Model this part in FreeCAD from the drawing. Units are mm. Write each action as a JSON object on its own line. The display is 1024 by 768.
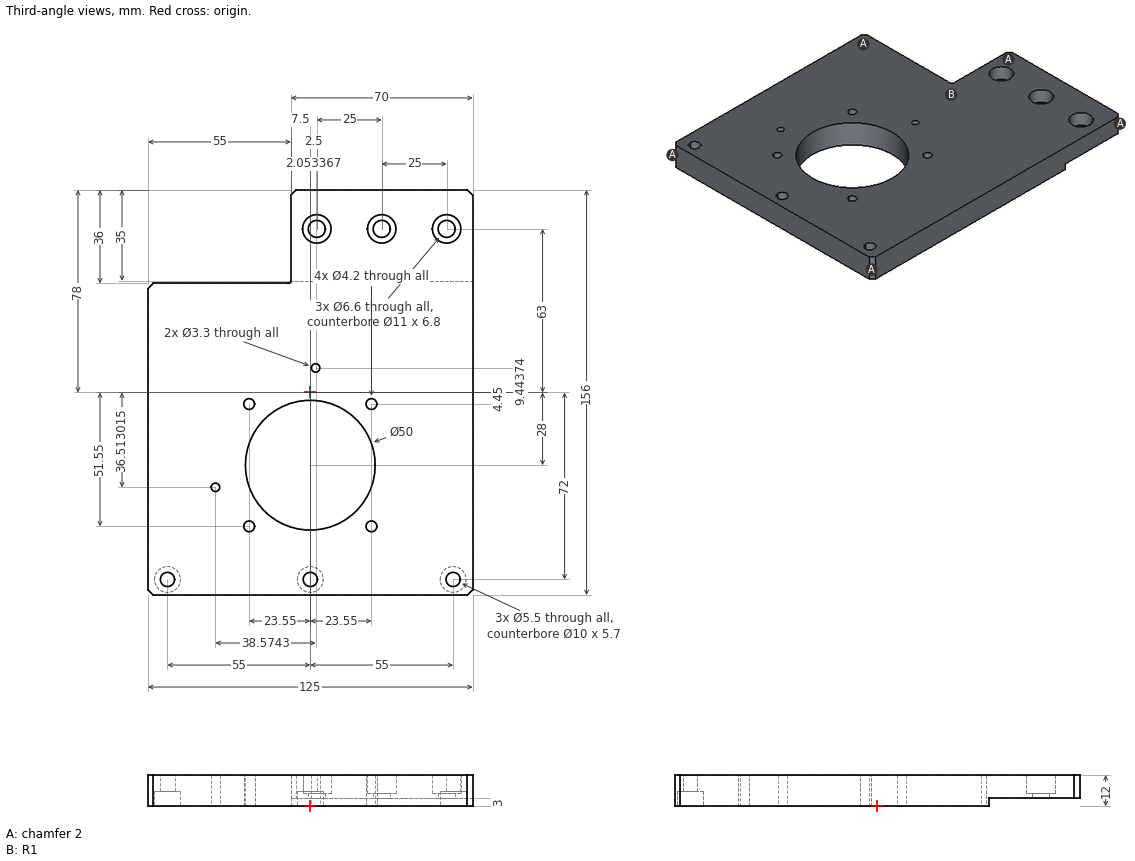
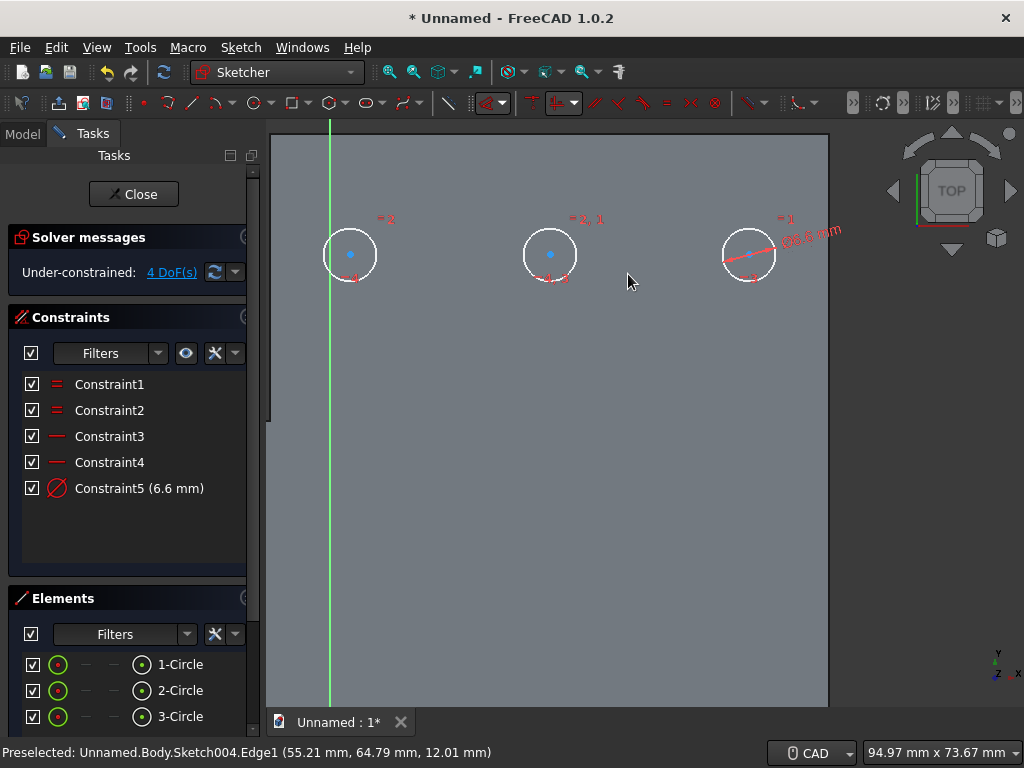
{"action": "left_click", "coordinate": [749, 255]}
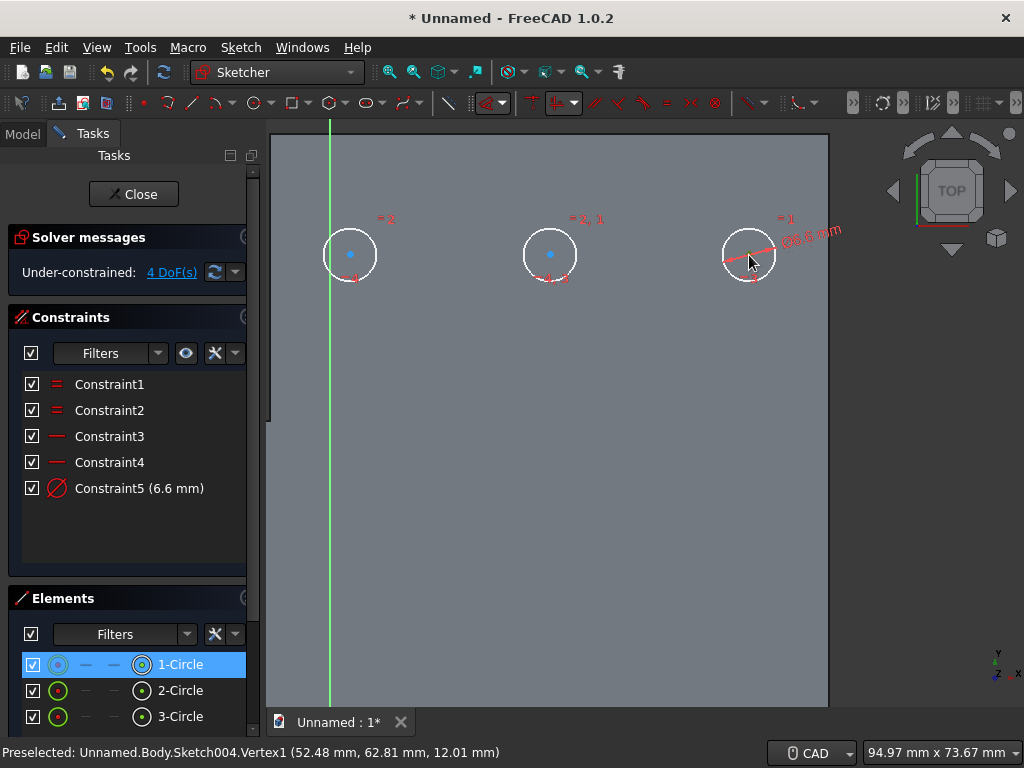
{"action": "left_click", "coordinate": [504, 104]}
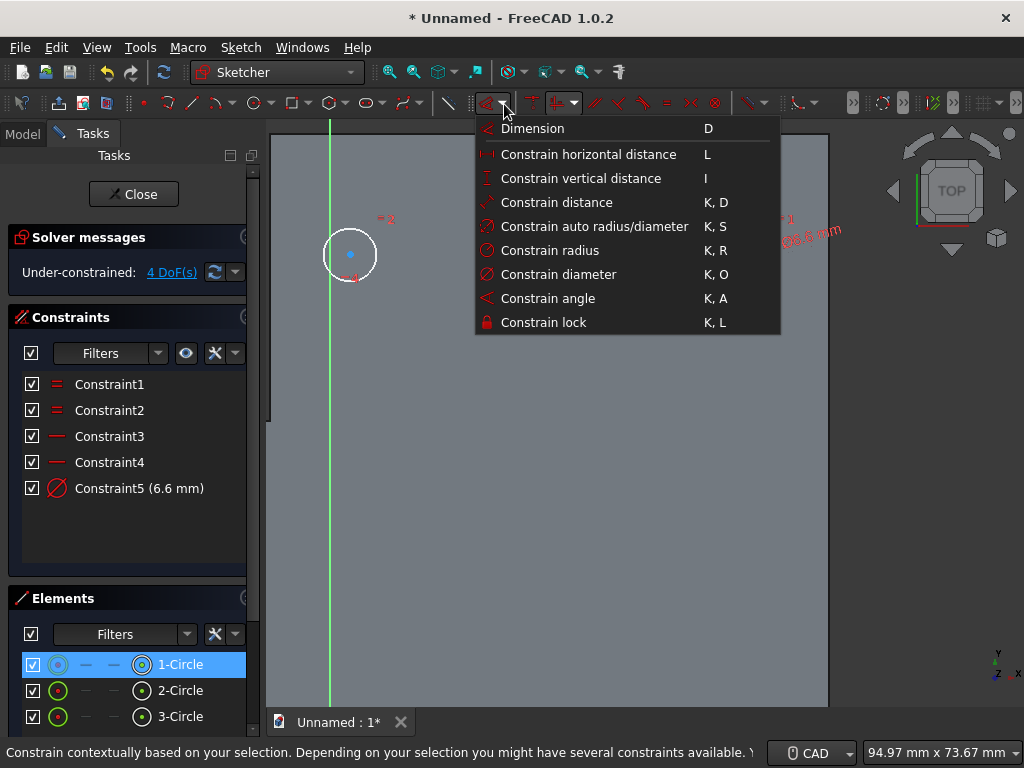
{"action": "left_click", "coordinate": [628, 178]}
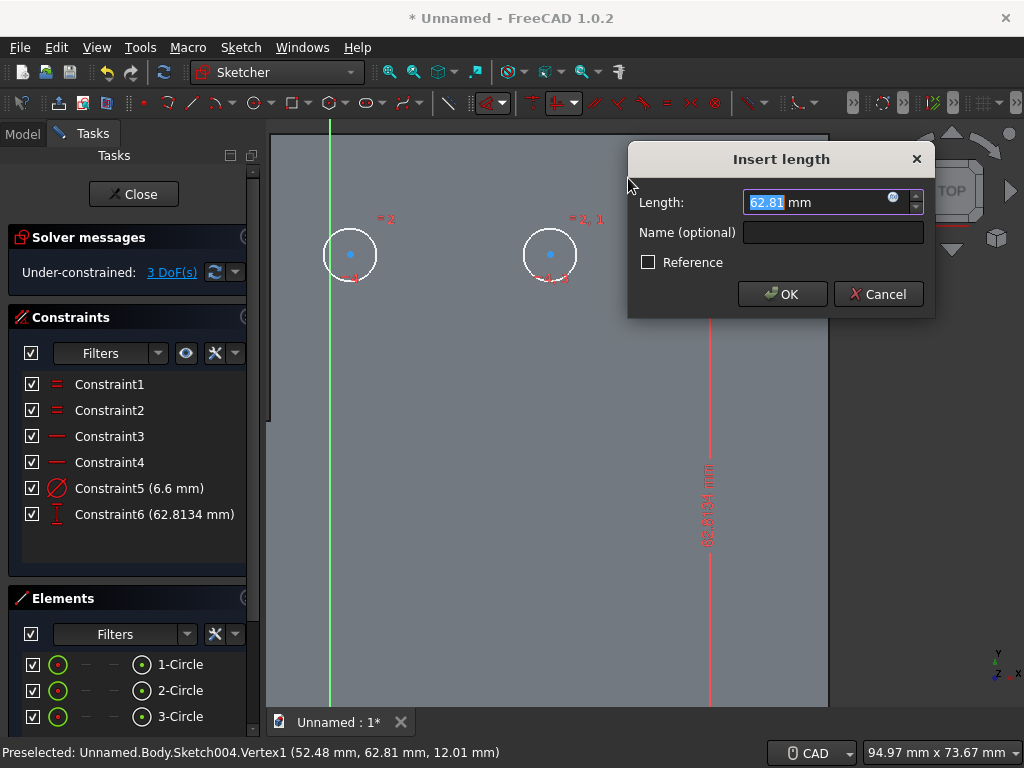
{"action": "type", "text": "63"}
{"action": "key", "text": "Return"}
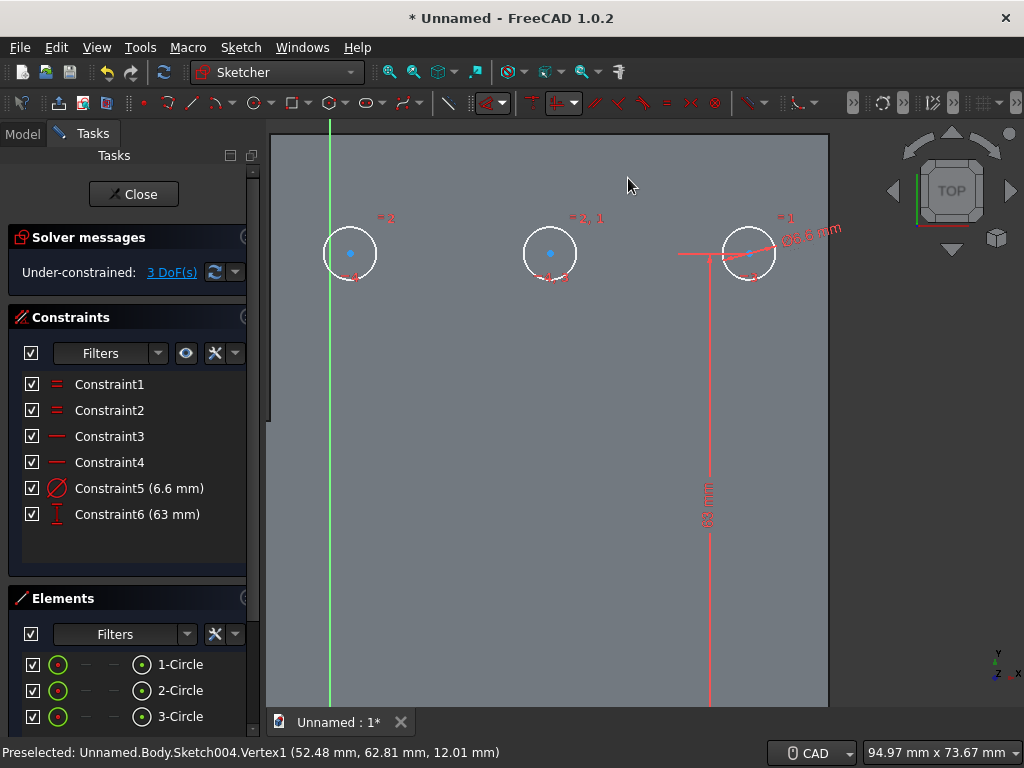
{"action": "scroll", "coordinate": [350, 254], "scroll_direction": "up", "scroll_amount": 4}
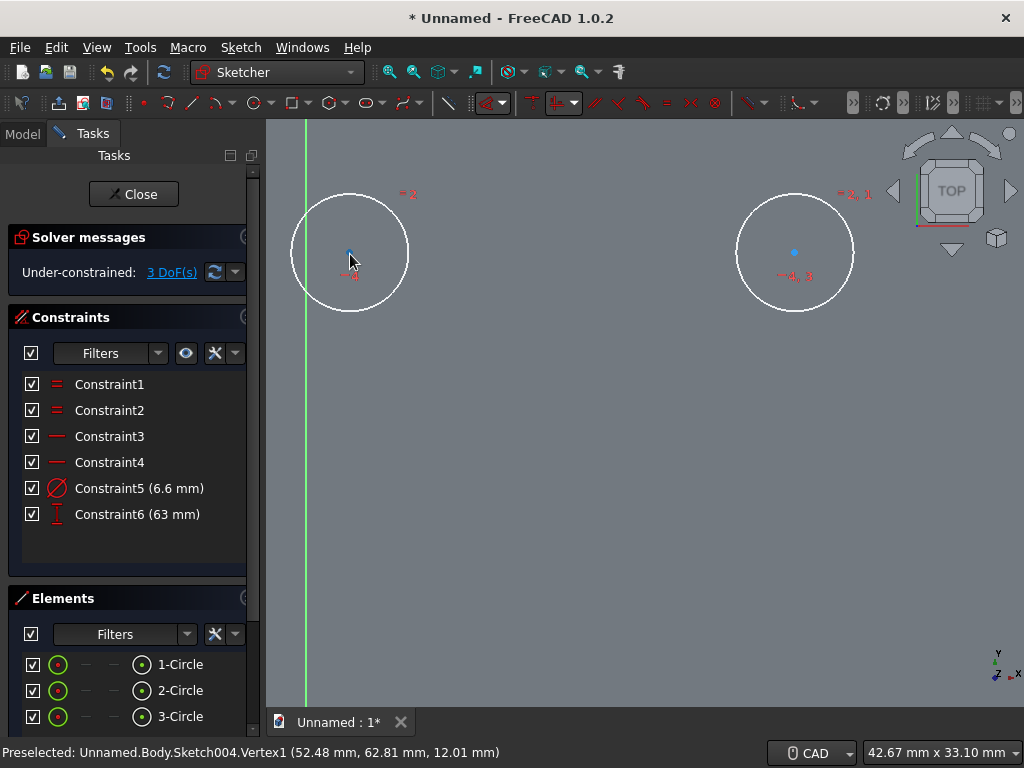
{"action": "left_click", "coordinate": [350, 253]}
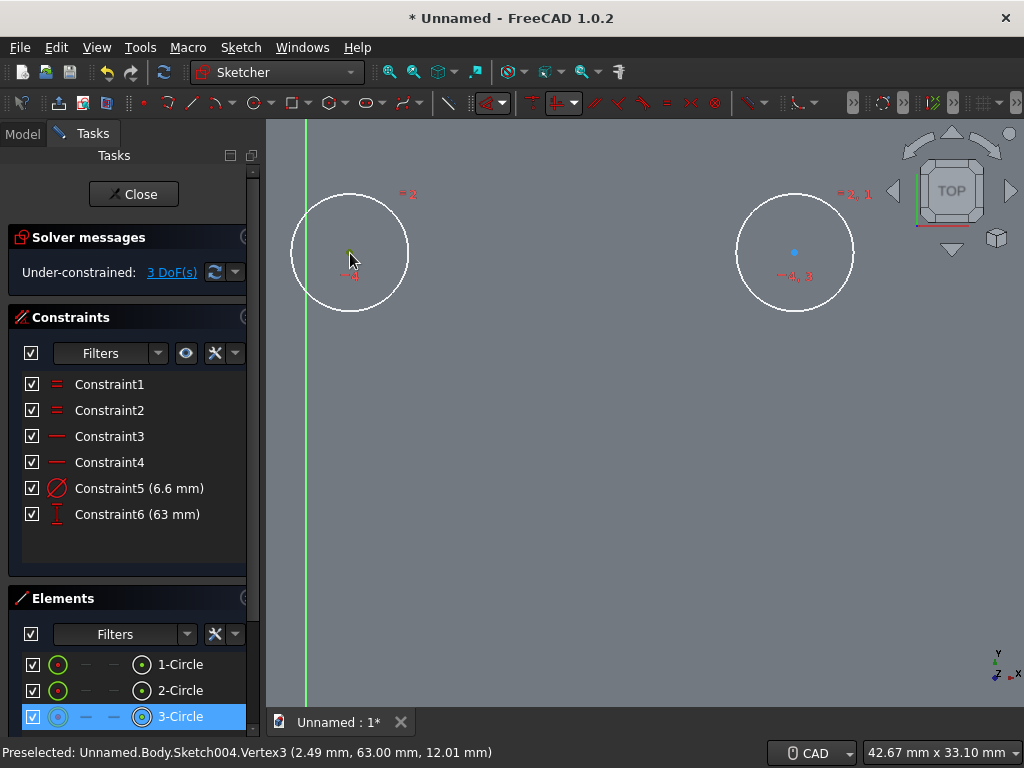
{"action": "left_click", "coordinate": [504, 104]}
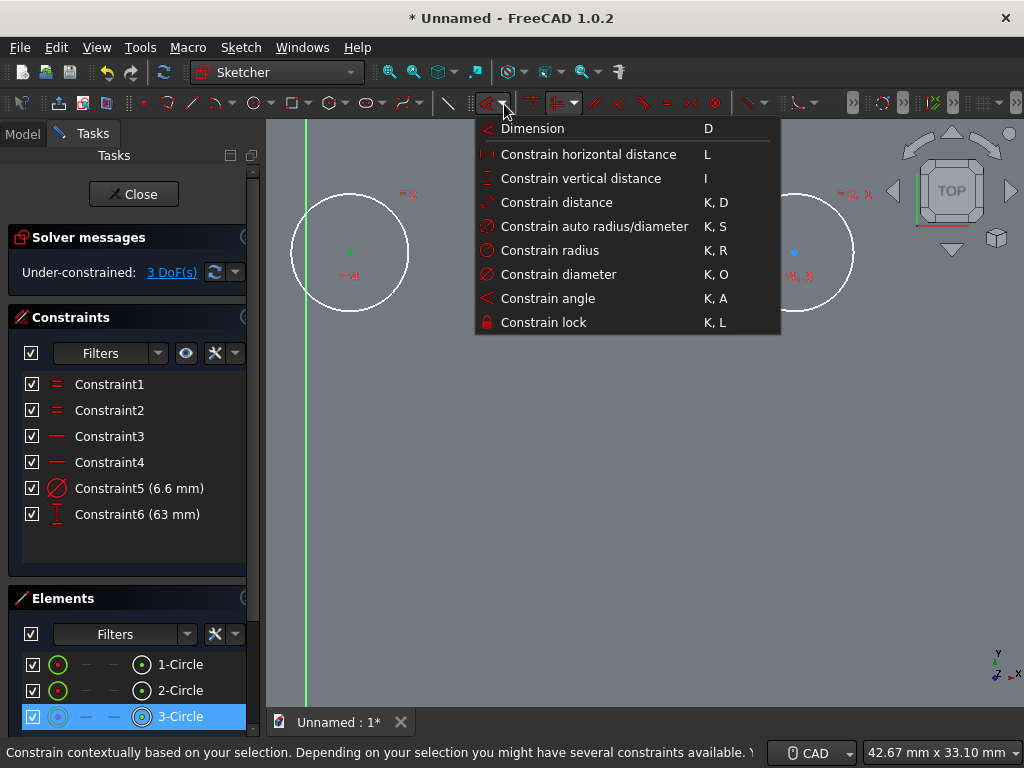
{"action": "left_click", "coordinate": [628, 154]}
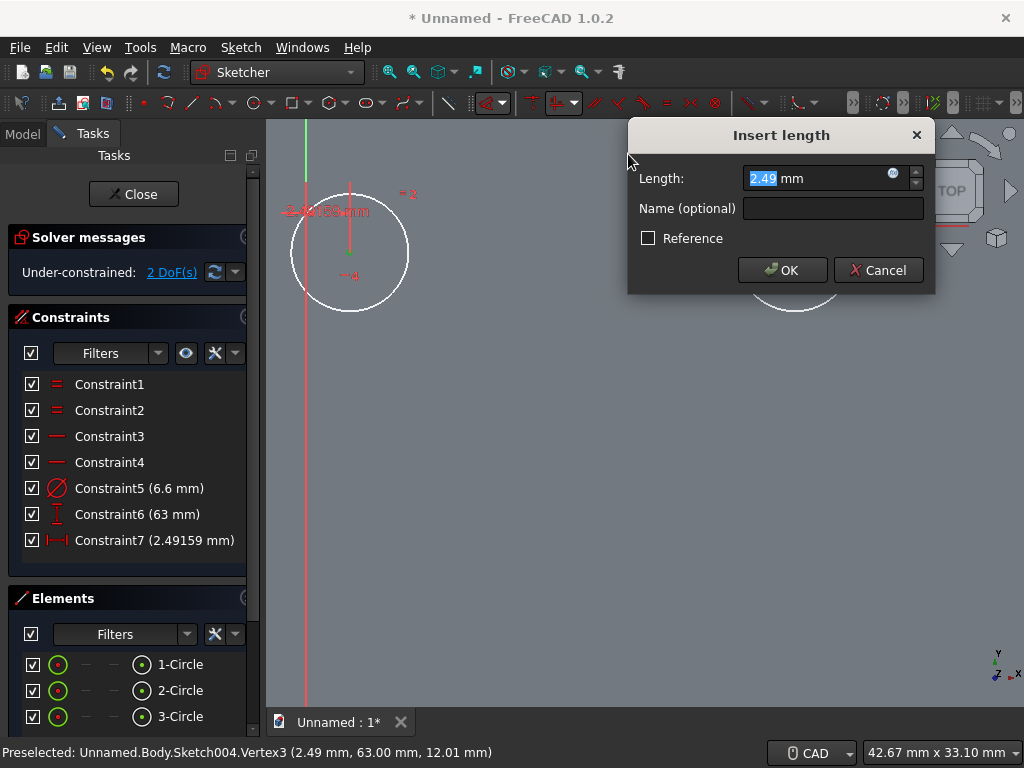
{"action": "type", "text": "2.5"}
{"action": "key", "text": "Return"}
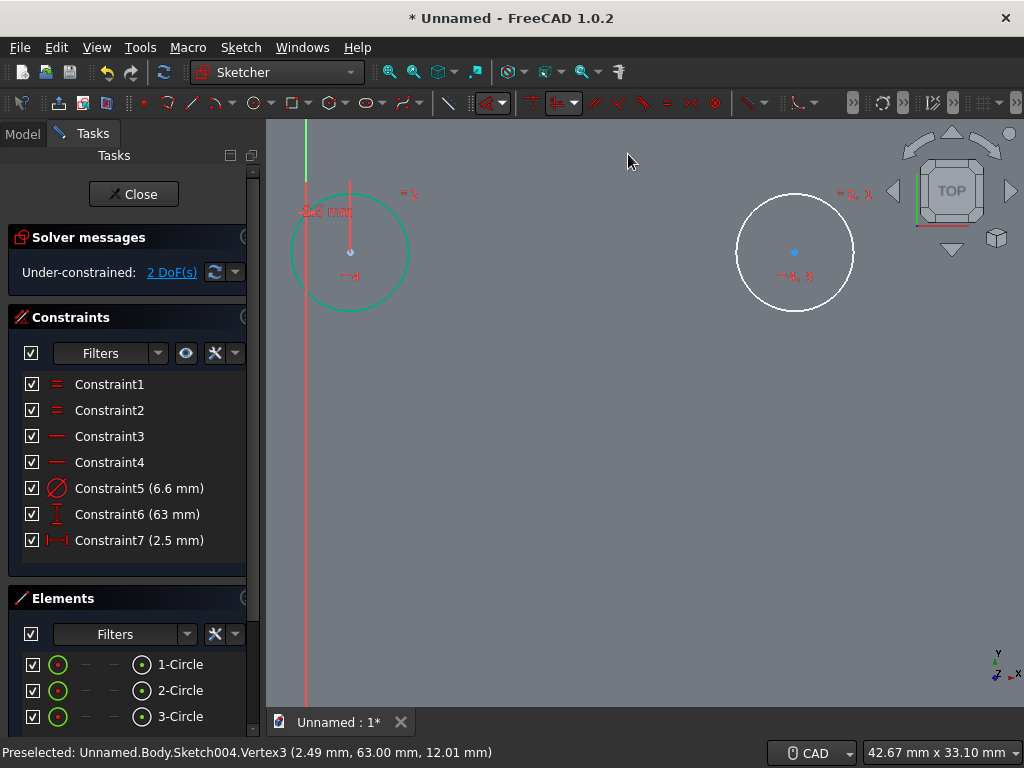
{"action": "scroll", "coordinate": [483, 254], "scroll_direction": "down", "scroll_amount": 6}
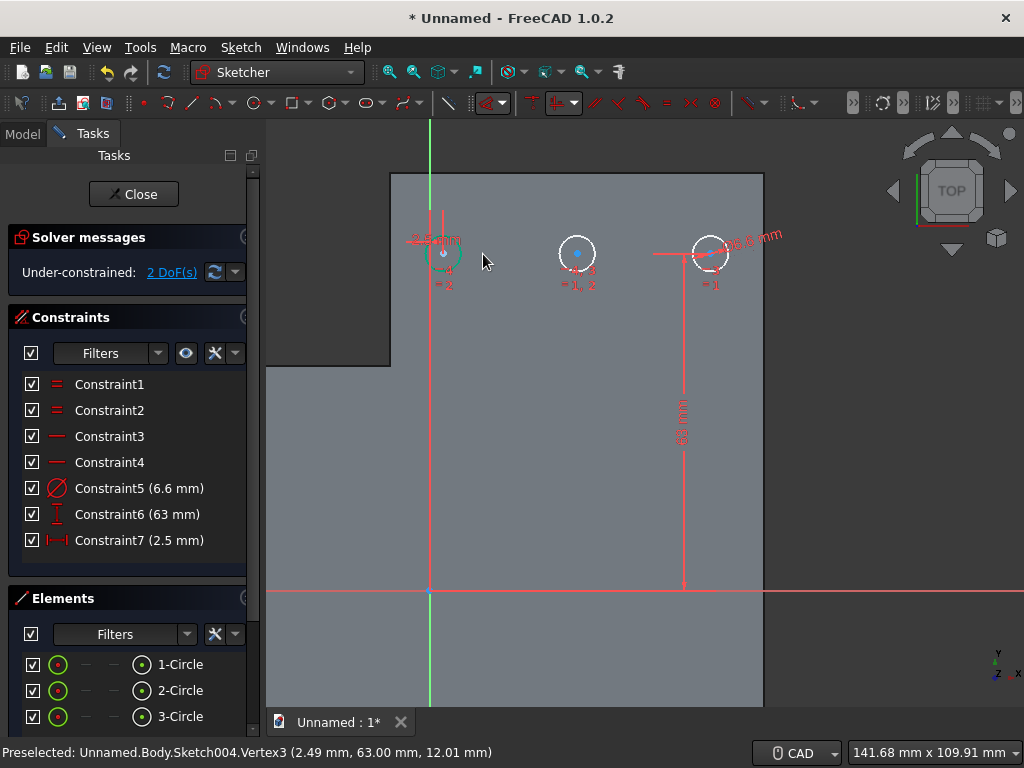
{"action": "left_click", "coordinate": [711, 254]}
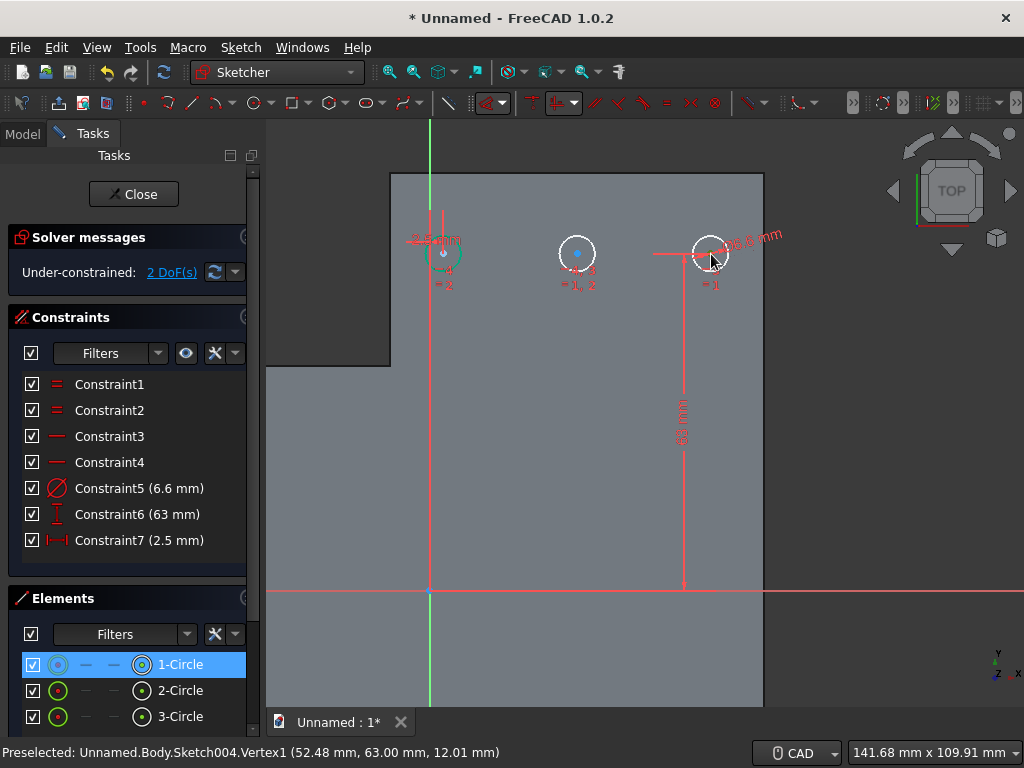
{"action": "left_click", "coordinate": [577, 254]}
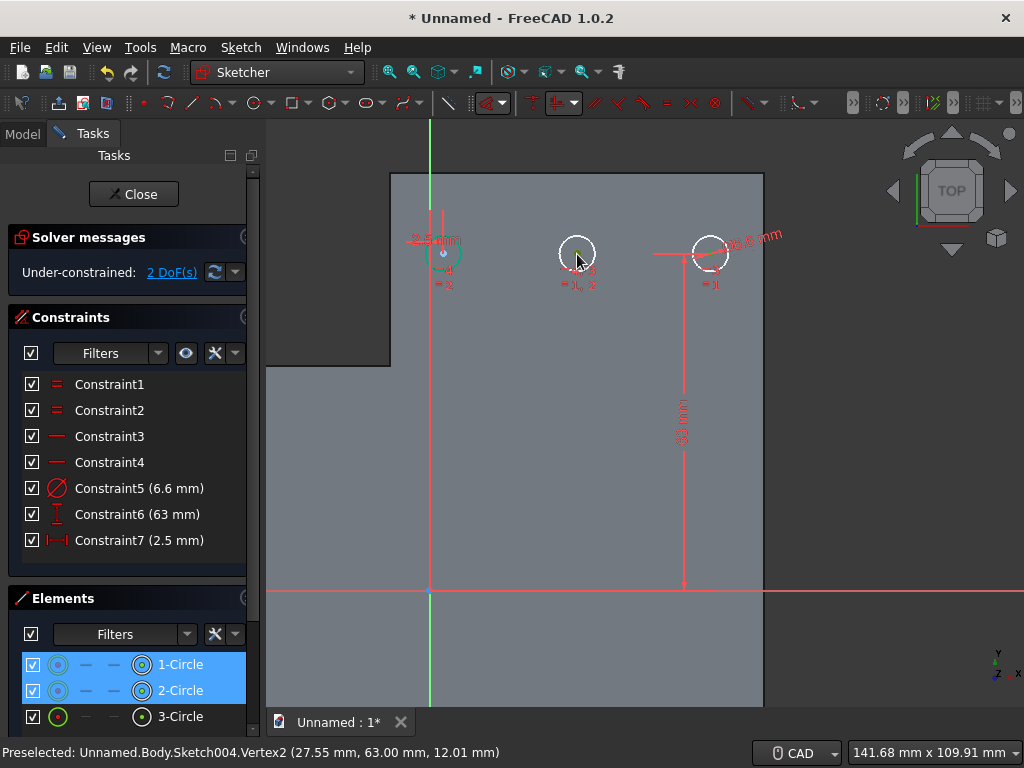
{"action": "left_click", "coordinate": [504, 104]}